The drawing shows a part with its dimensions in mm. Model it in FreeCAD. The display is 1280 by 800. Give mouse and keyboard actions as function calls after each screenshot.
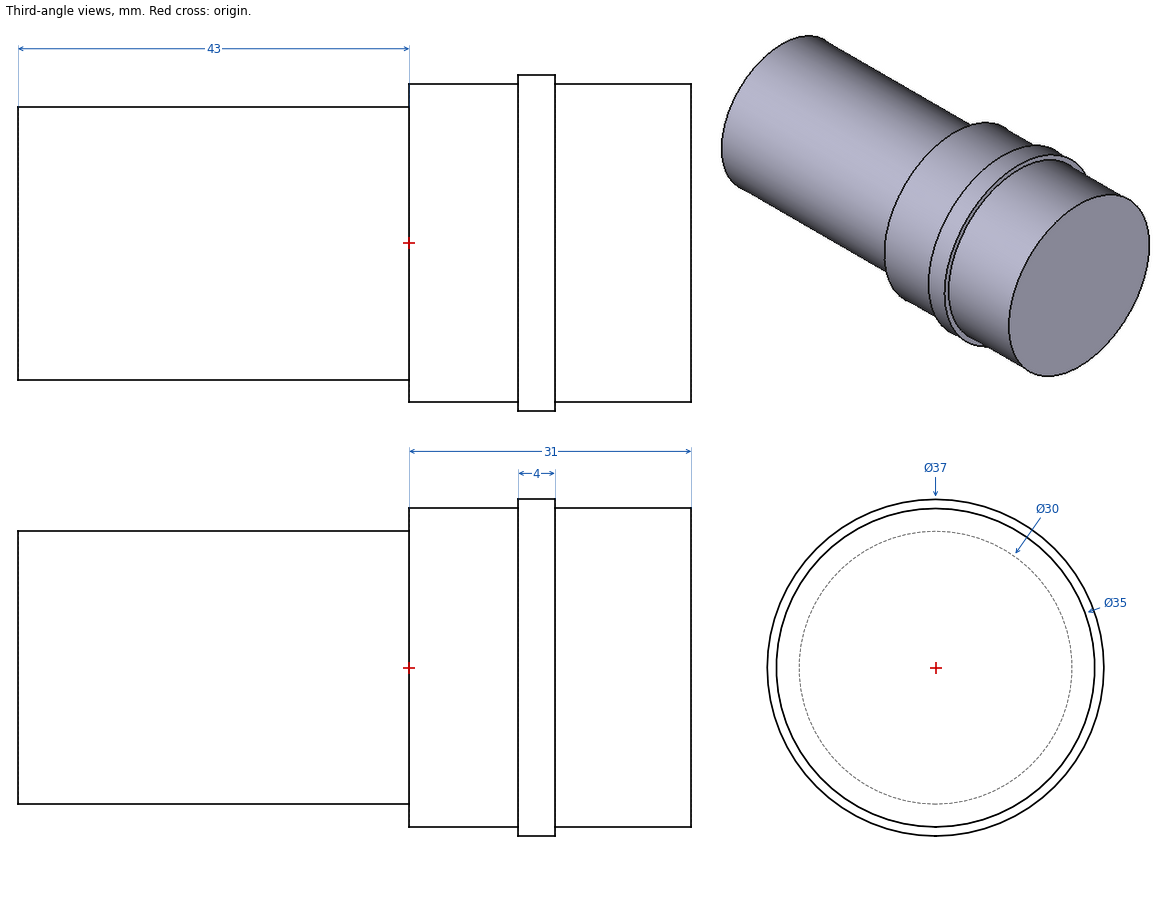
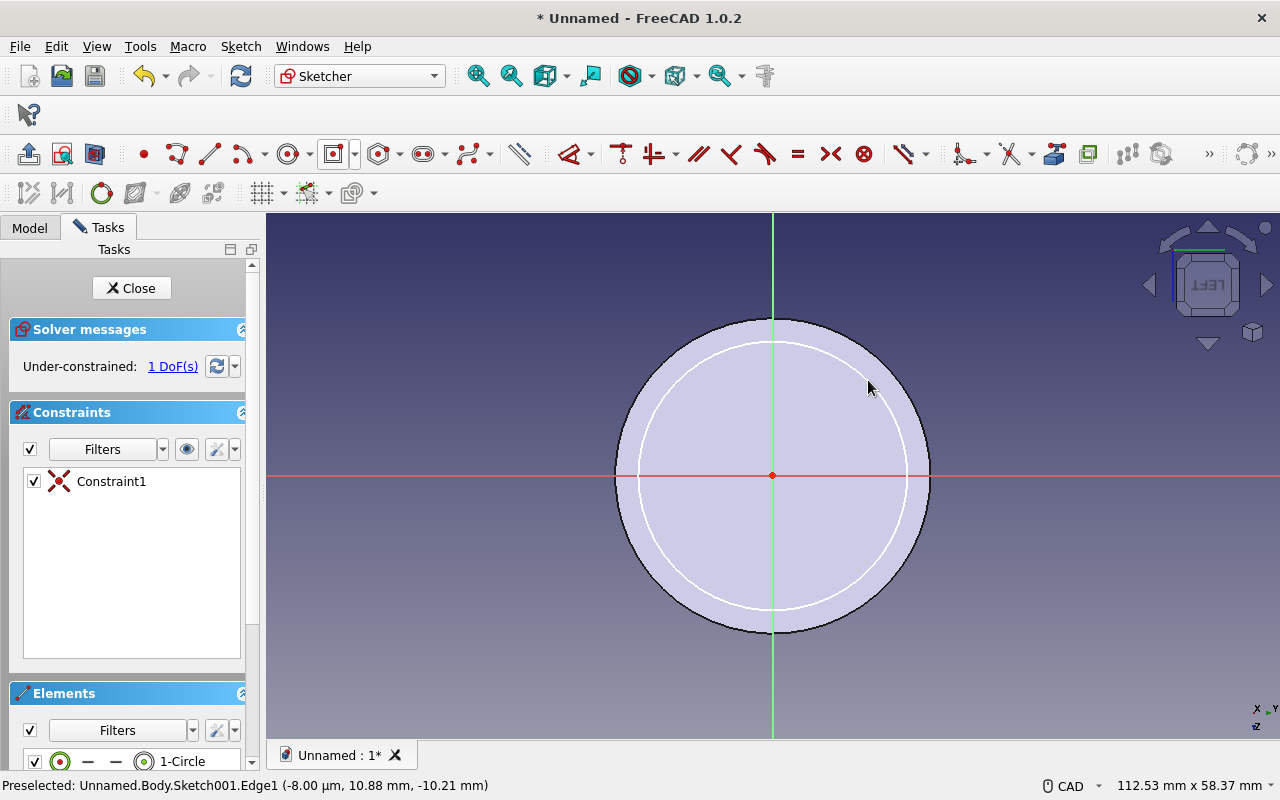
key(d)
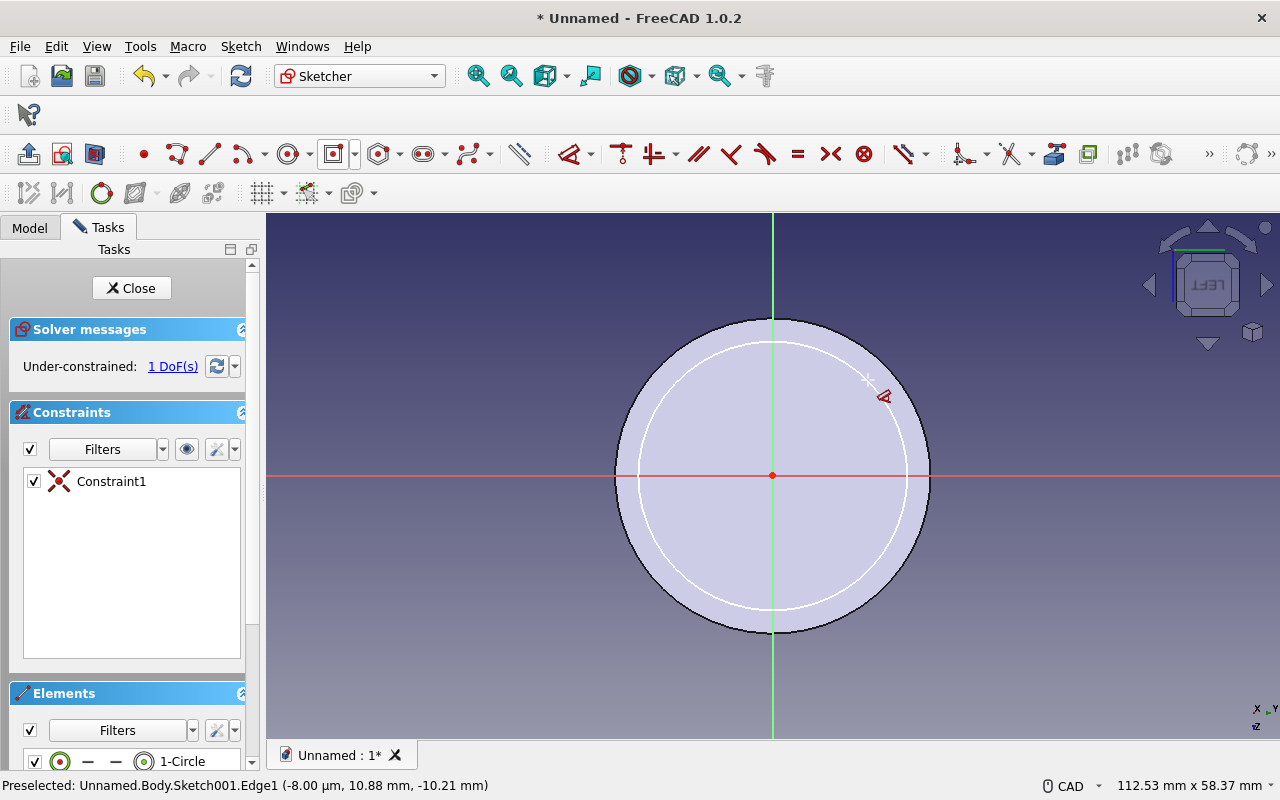
click(868, 381)
click(891, 358)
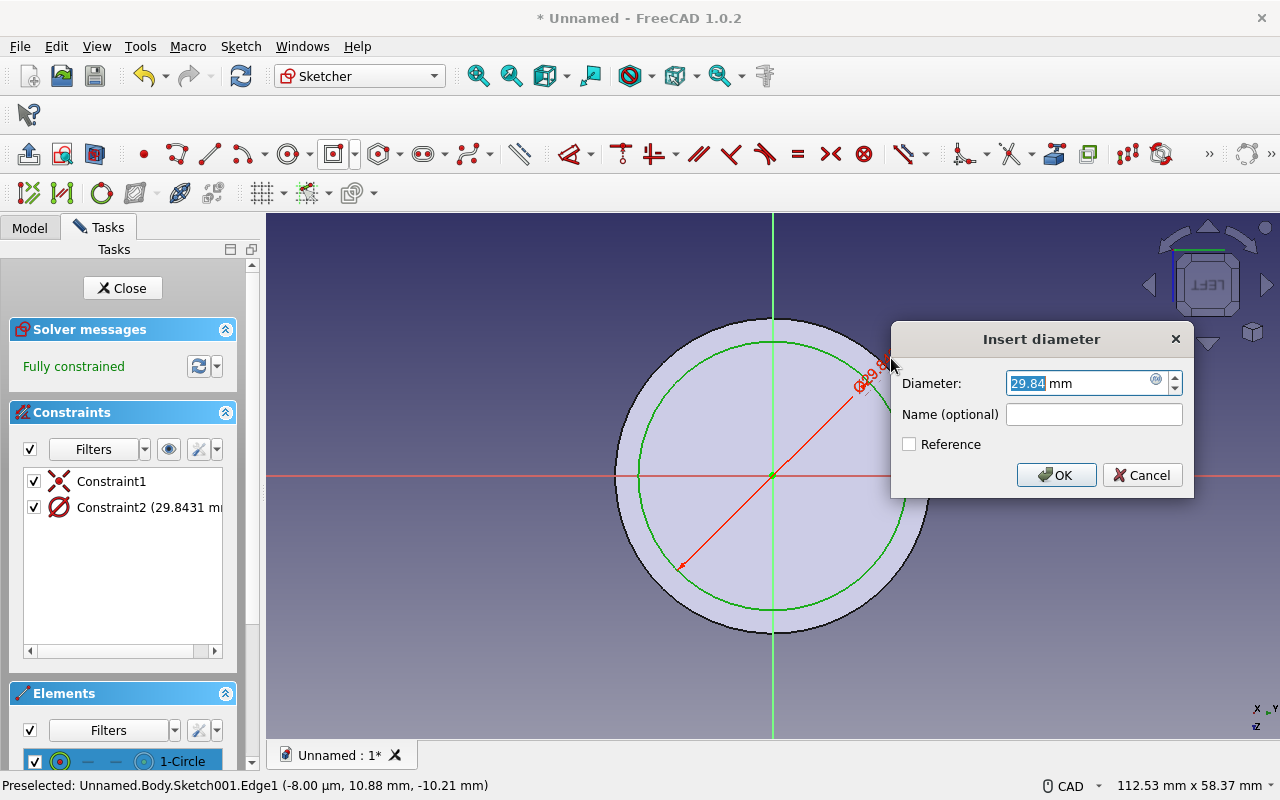
text(30)
key(Return)
key(Escape)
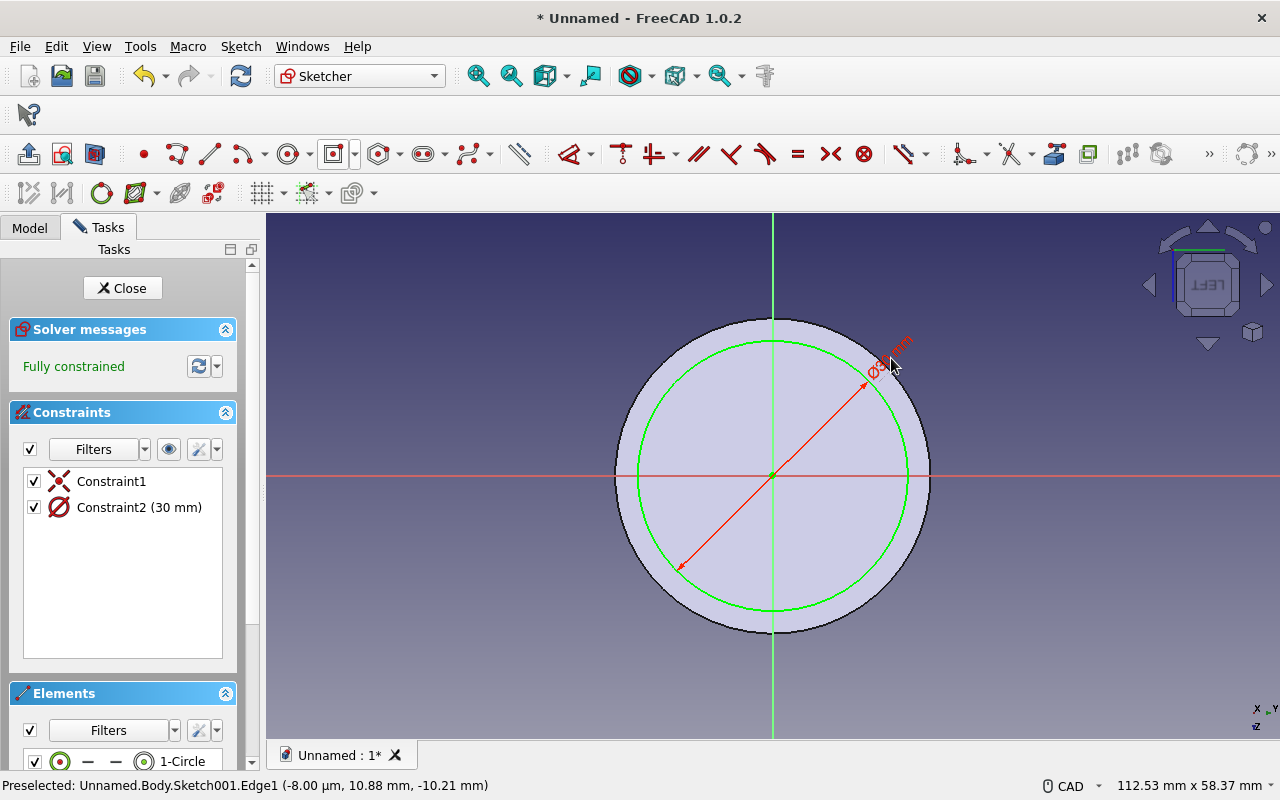
click(123, 288)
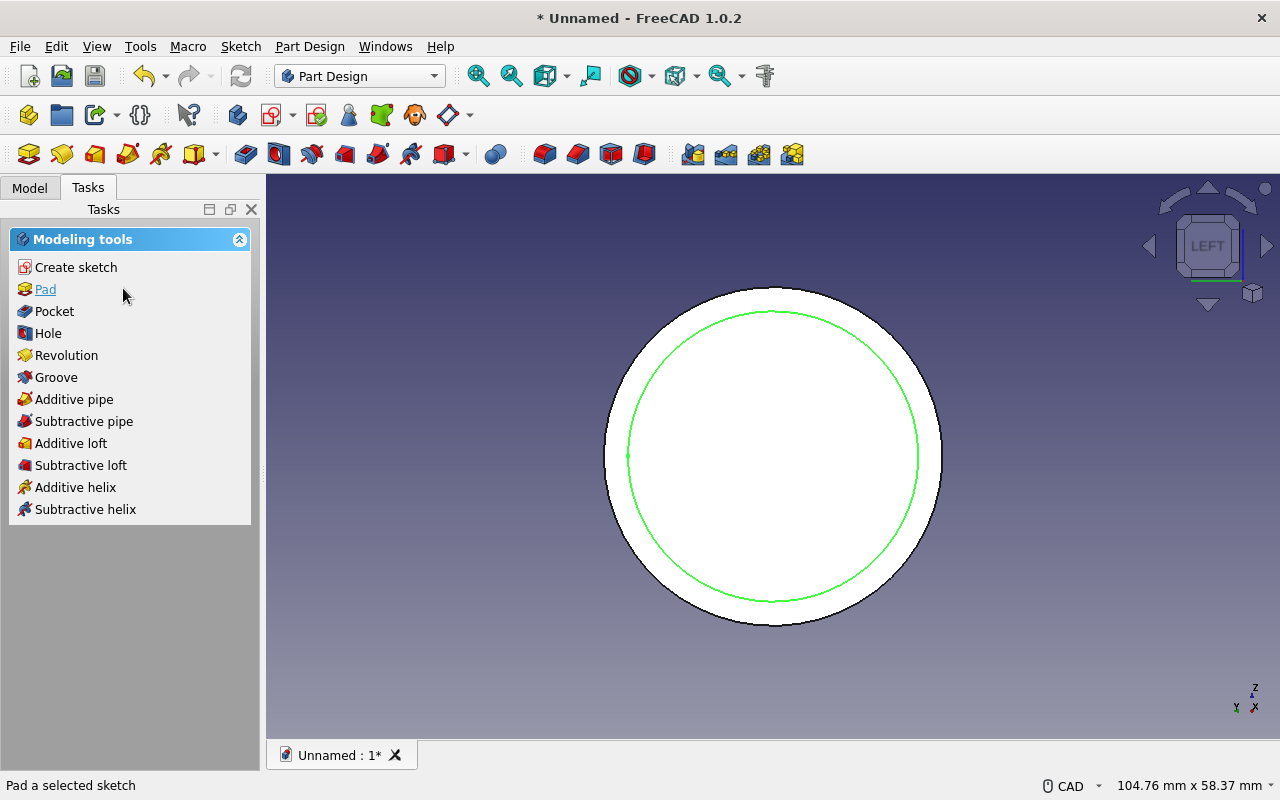
click(29, 154)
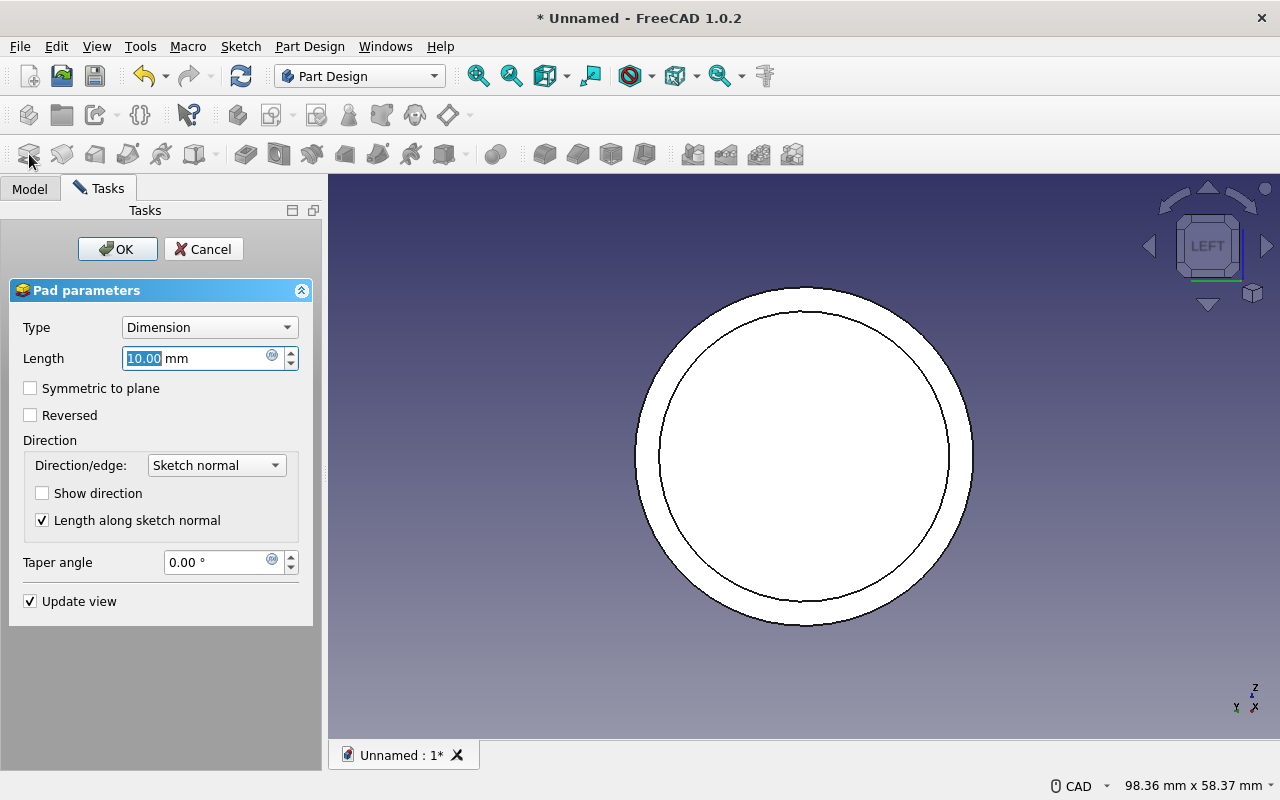
text(43)
key(Tab)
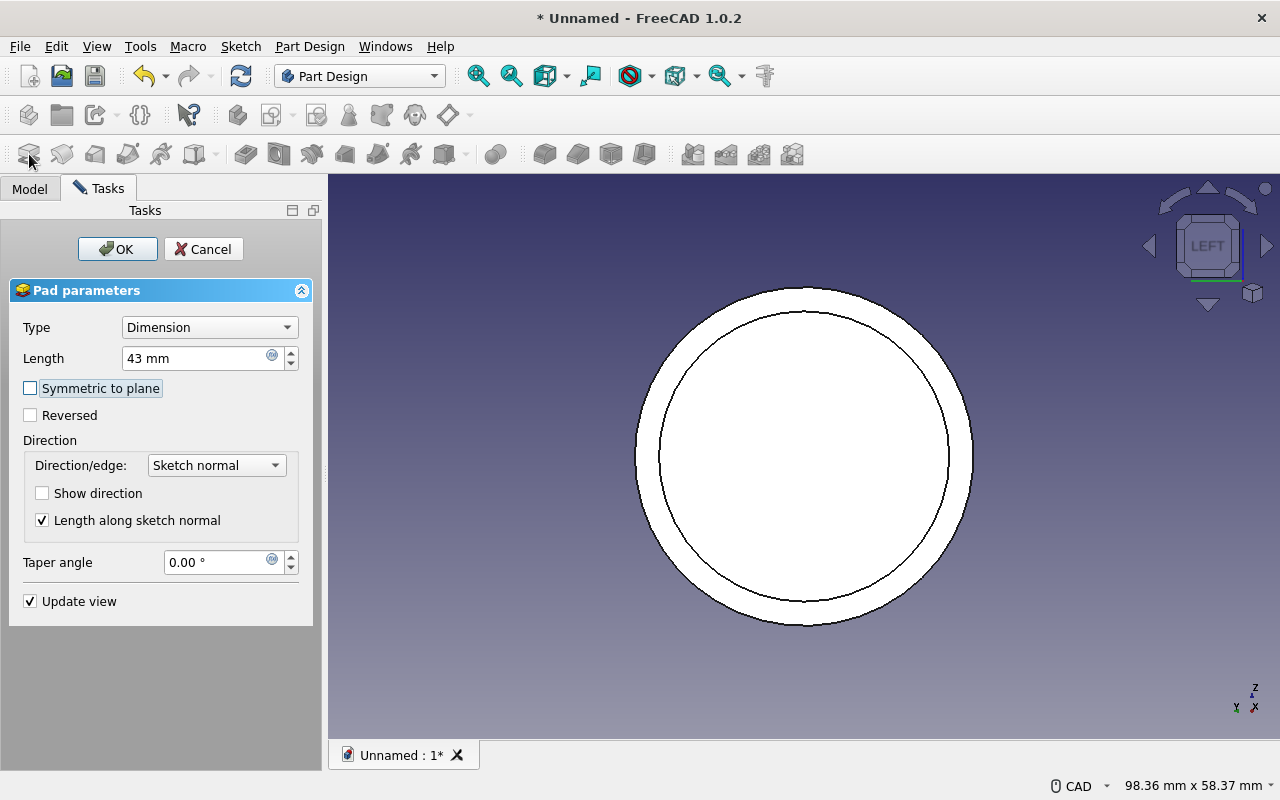
click(118, 249)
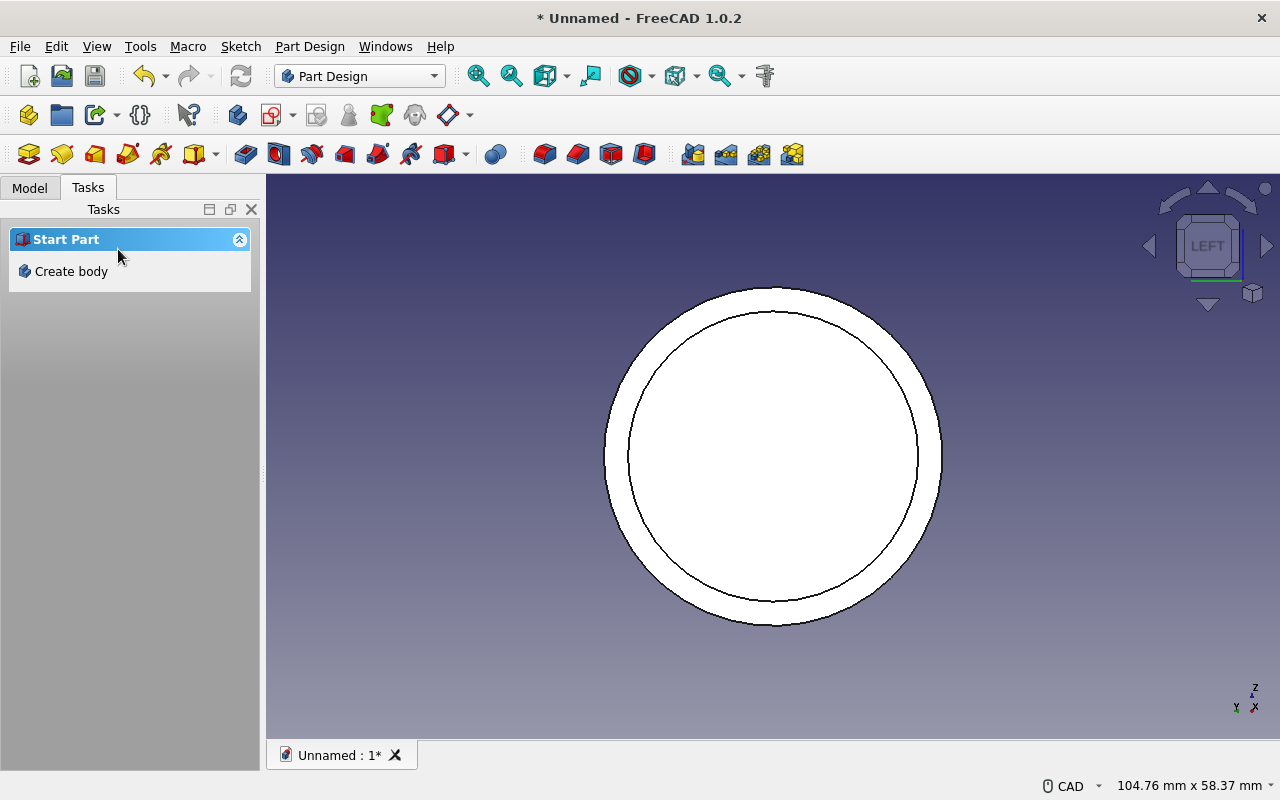
click(30, 188)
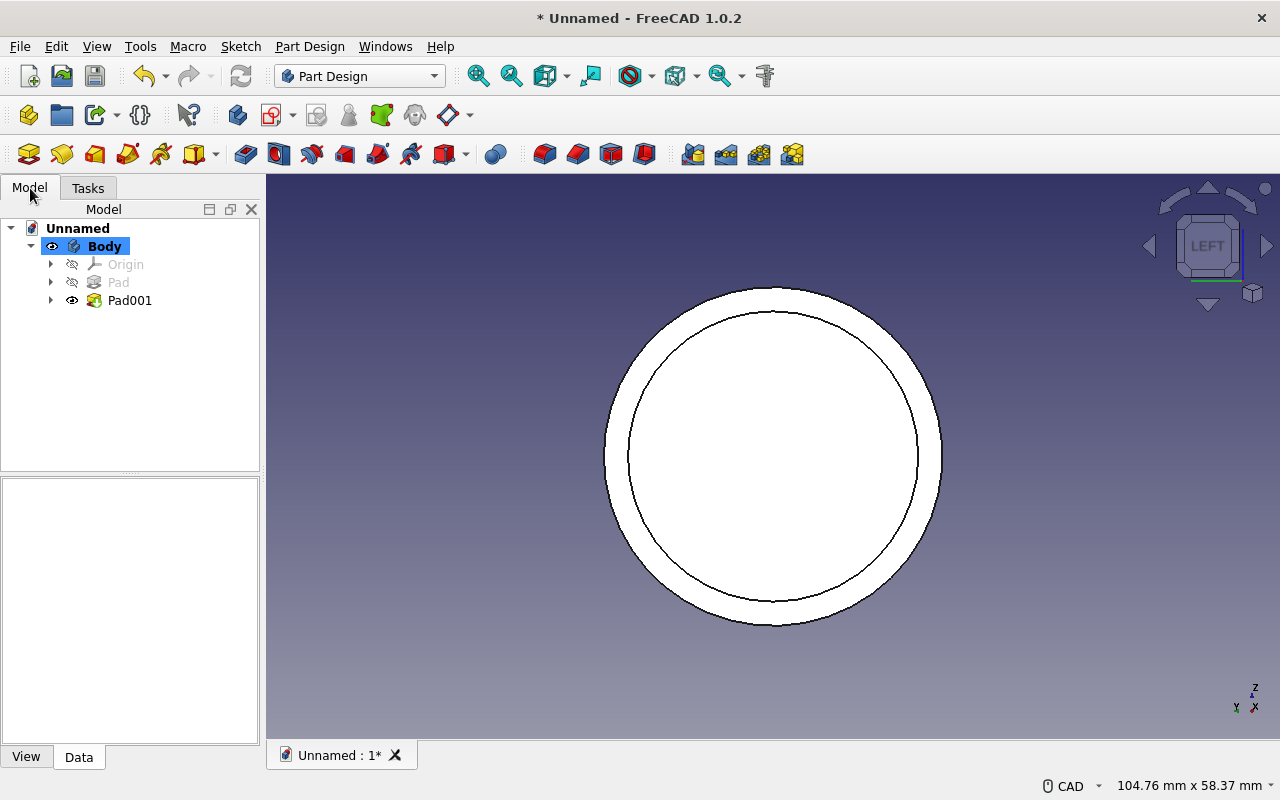
click(51, 264)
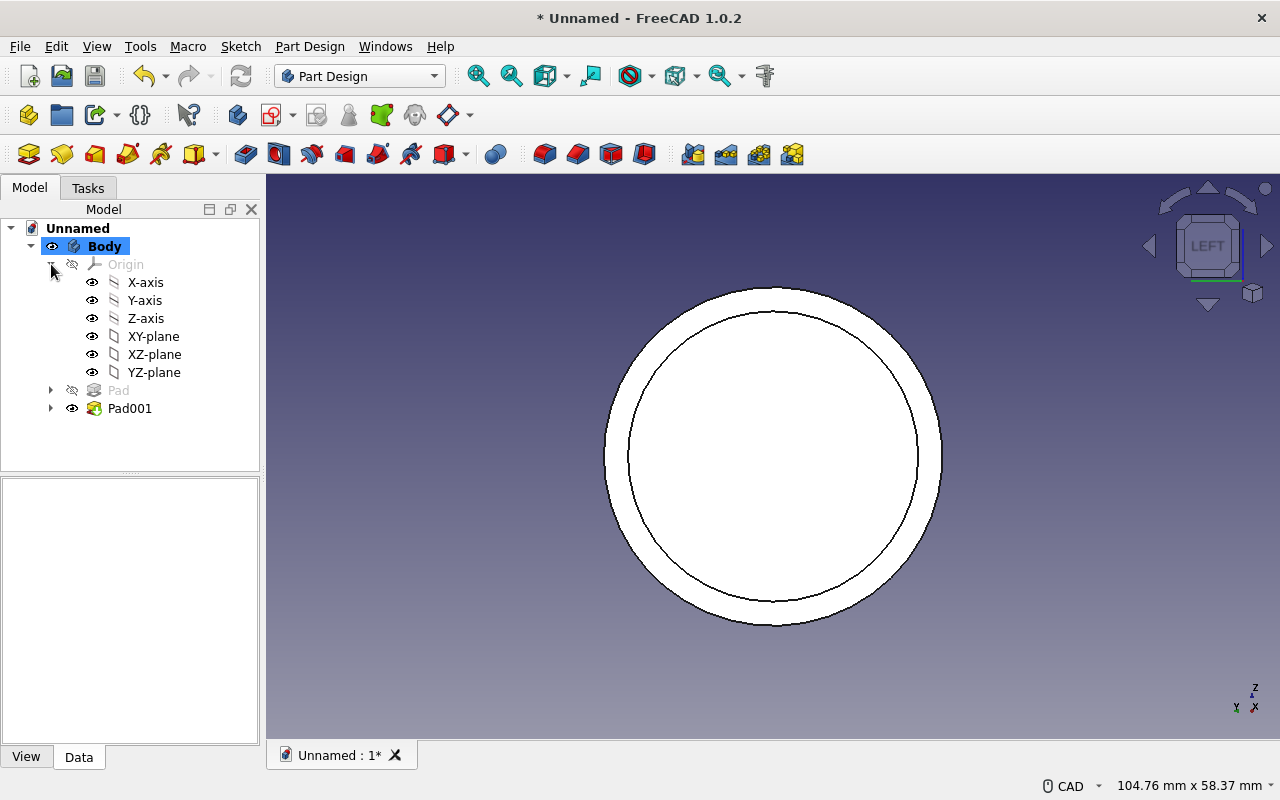
click(137, 372)